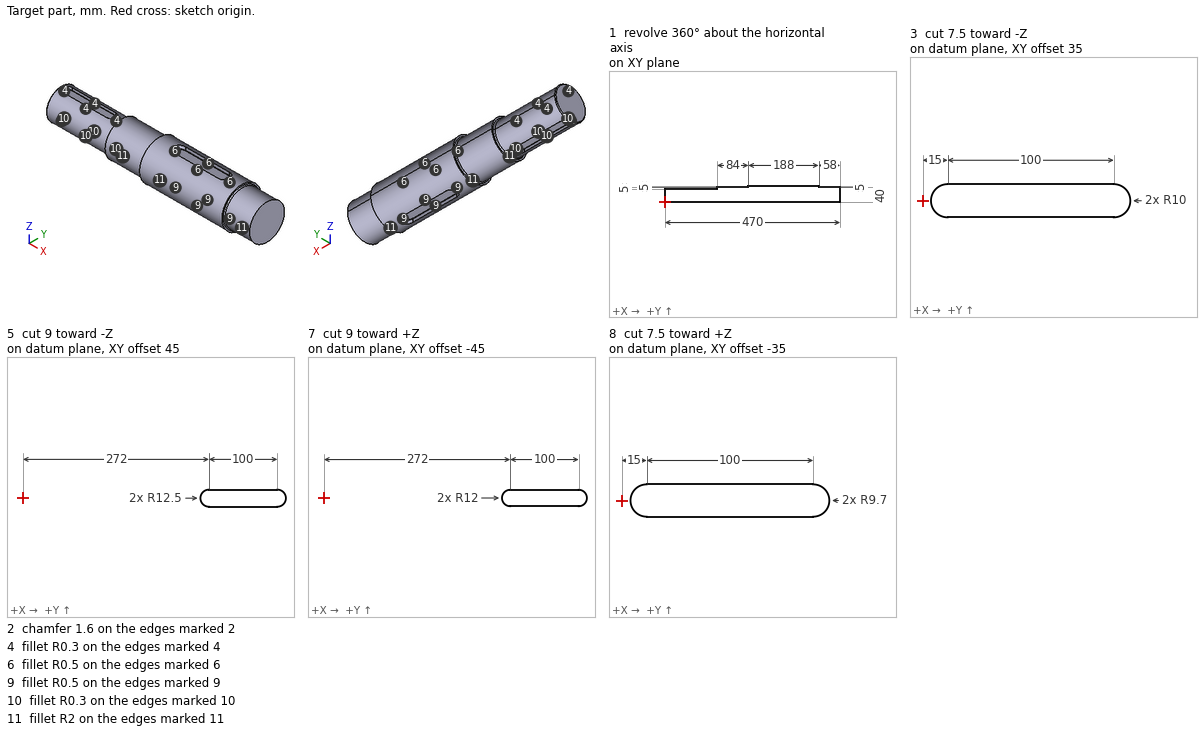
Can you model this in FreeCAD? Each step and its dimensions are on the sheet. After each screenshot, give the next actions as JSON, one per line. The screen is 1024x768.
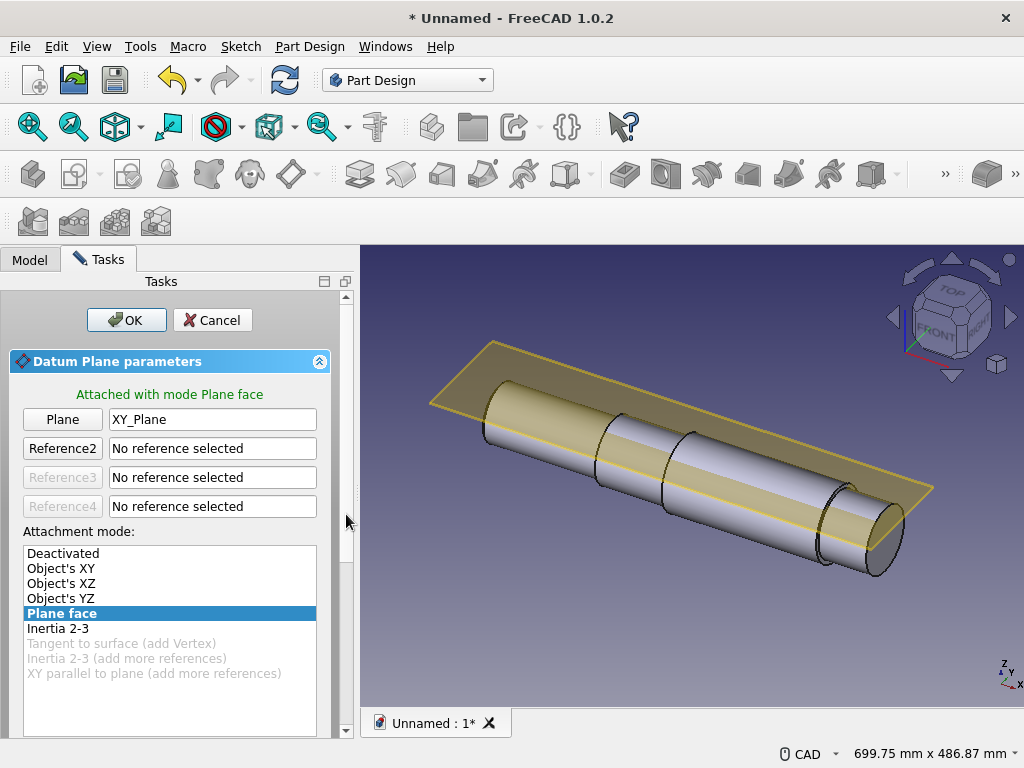
{"action": "left_click", "coordinate": [127, 320]}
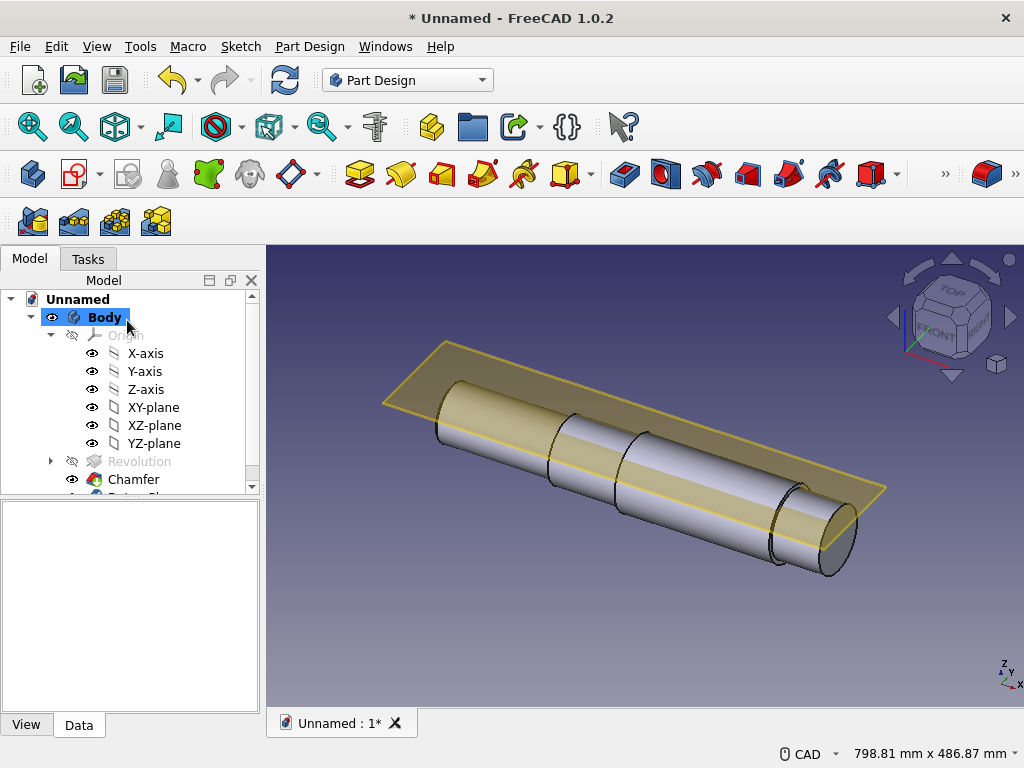
{"action": "scroll", "coordinate": [101, 385], "scroll_direction": "down", "scroll_amount": 3}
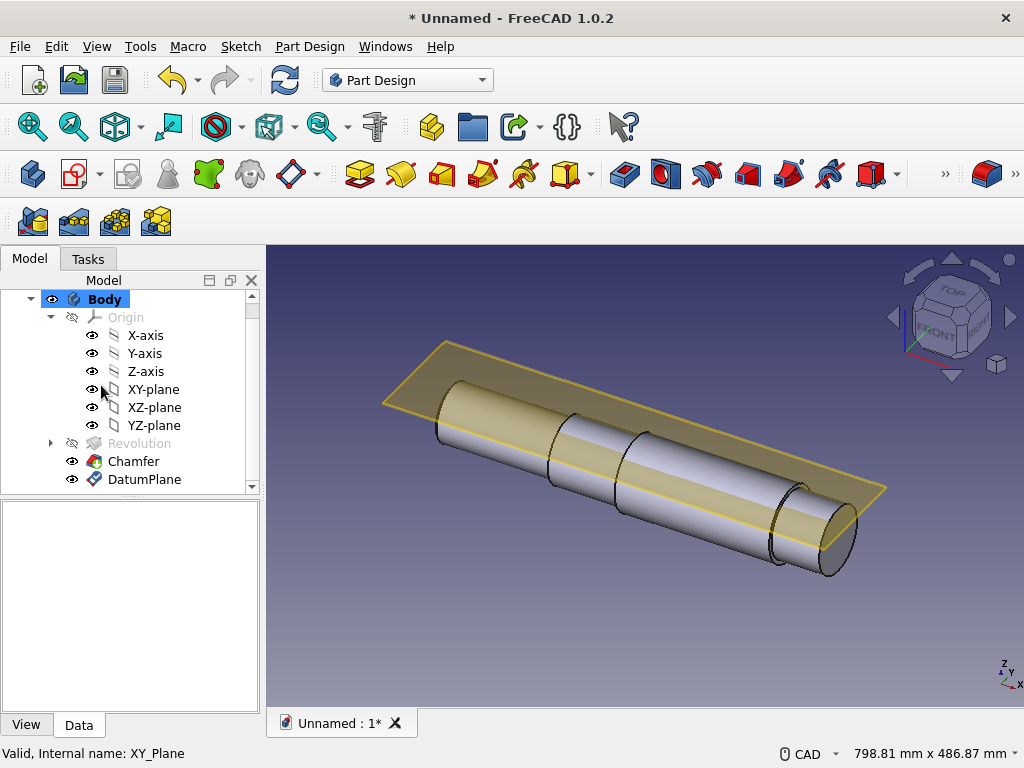
{"action": "left_click", "coordinate": [117, 479]}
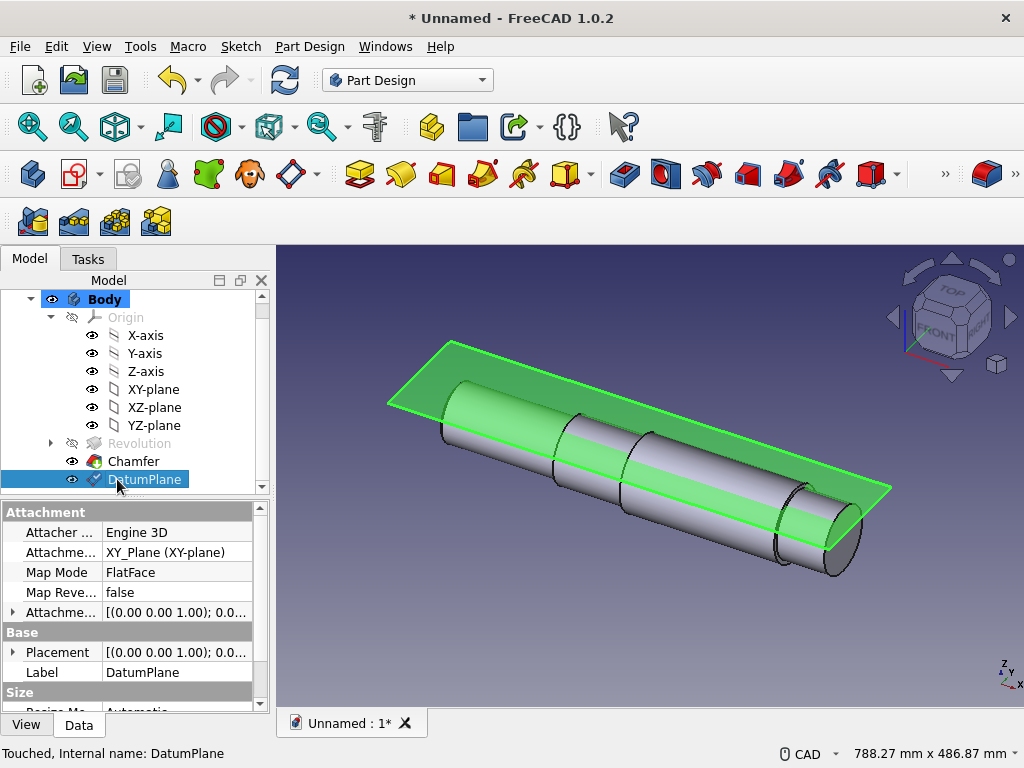
{"action": "left_click", "coordinate": [74, 174]}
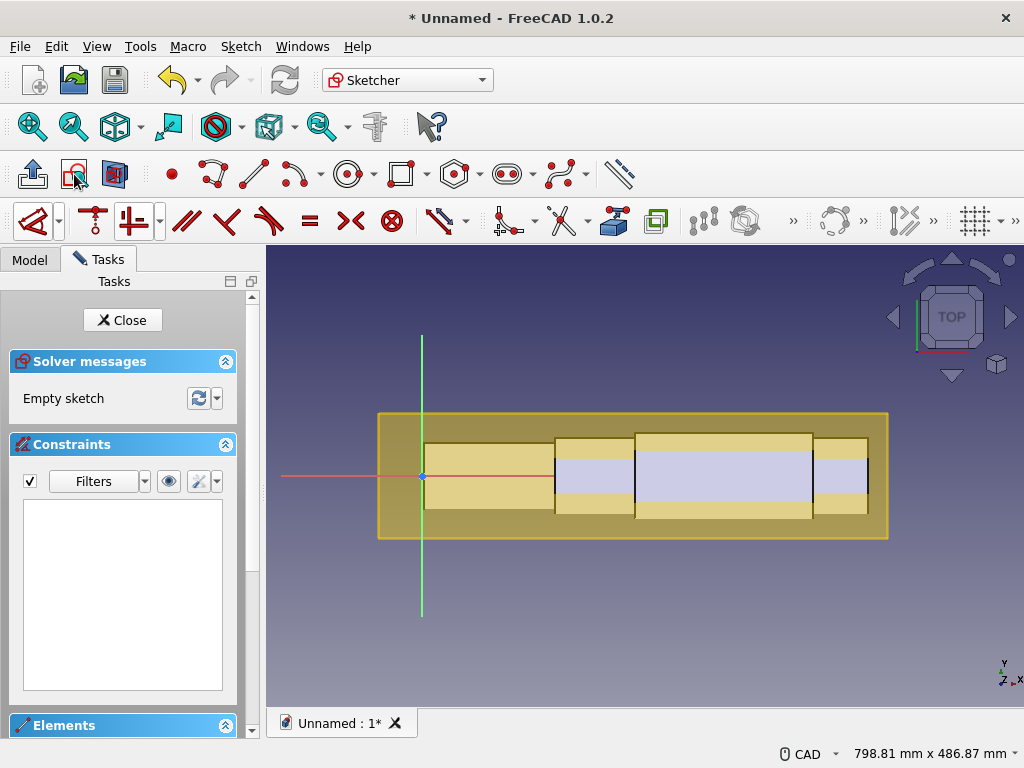
{"action": "left_click", "coordinate": [115, 174]}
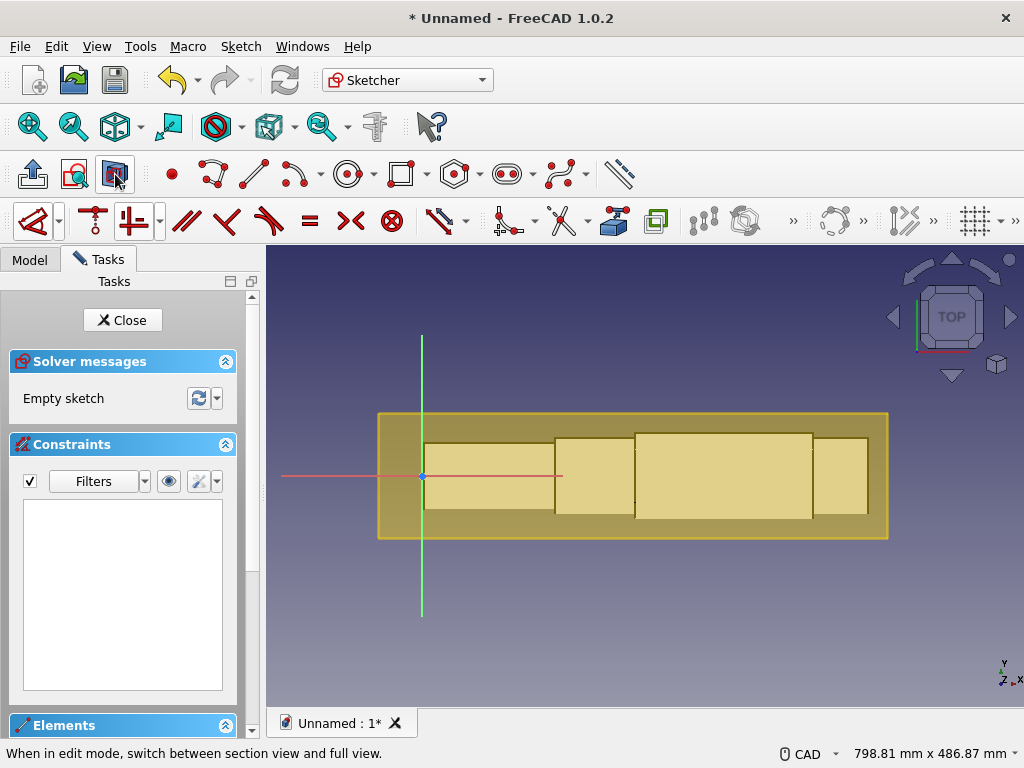
{"action": "scroll", "coordinate": [440, 476], "scroll_direction": "up", "scroll_amount": 6}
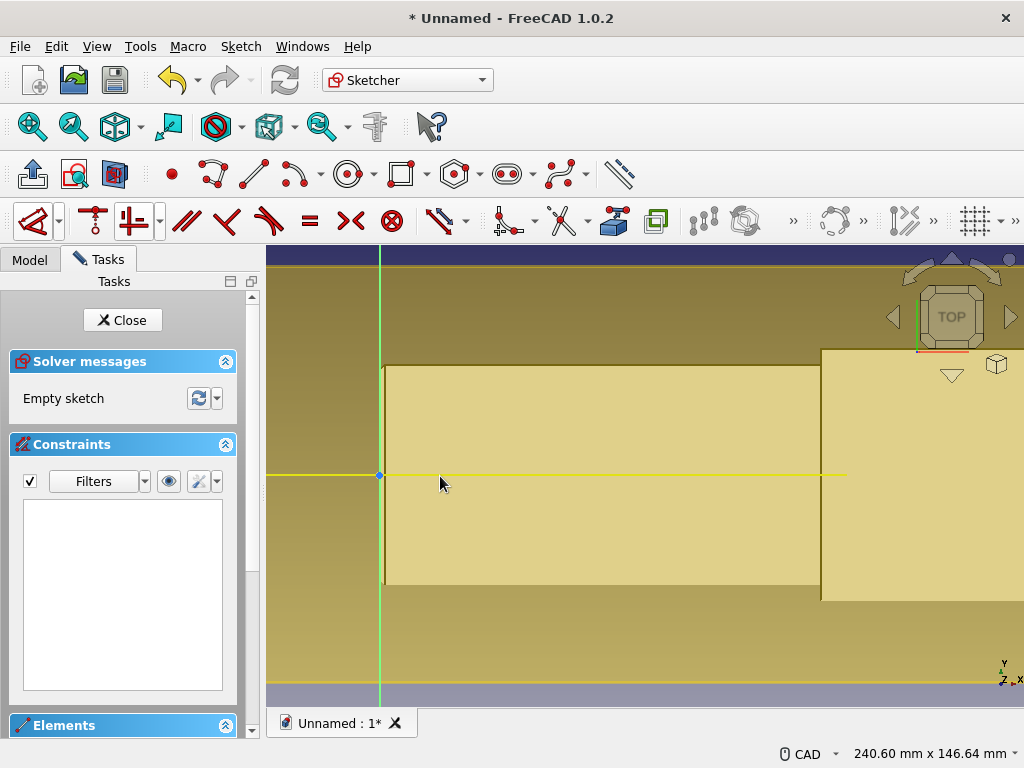
{"action": "left_click", "coordinate": [506, 174]}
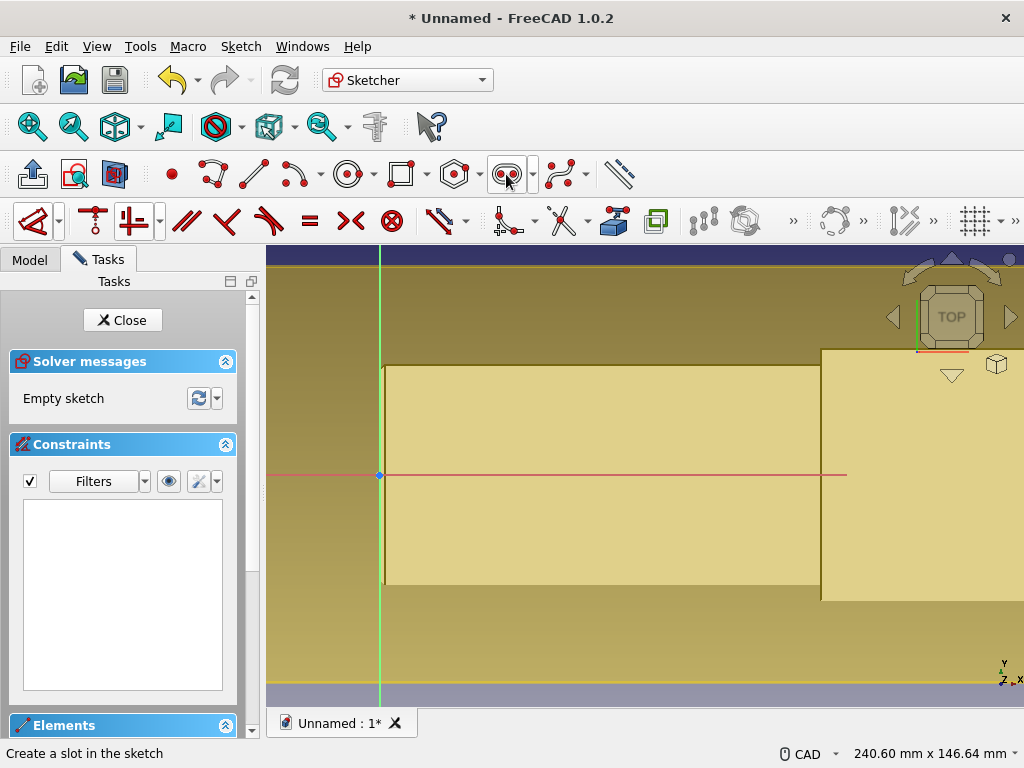
{"action": "left_click", "coordinate": [427, 475]}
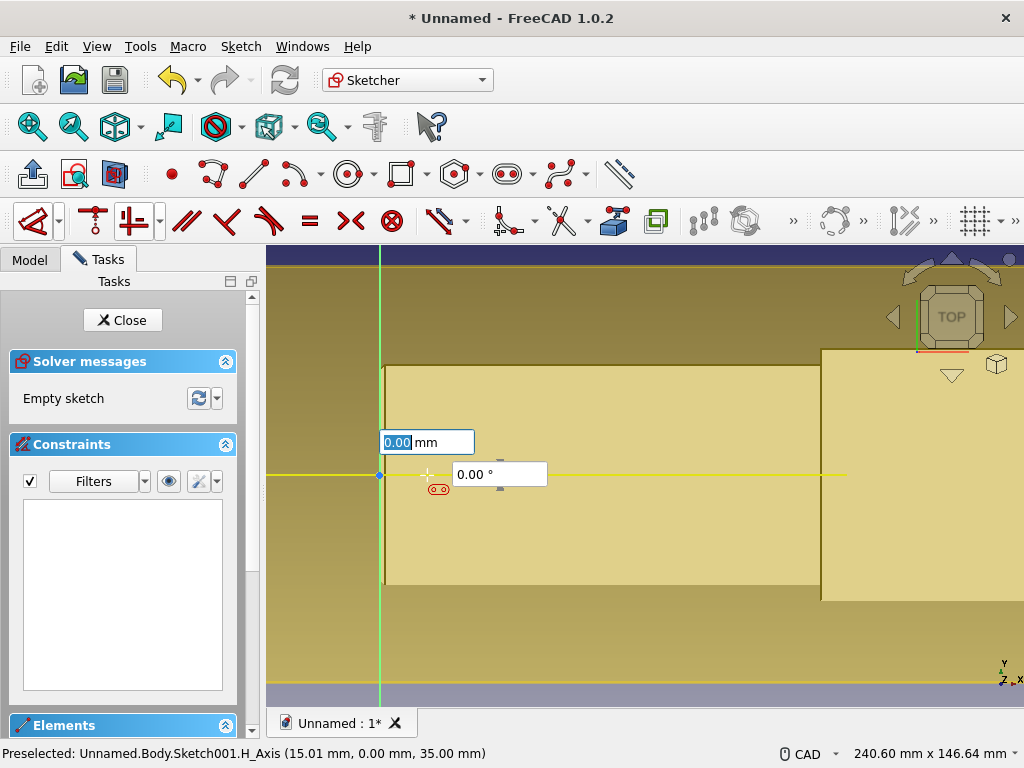
{"action": "left_click", "coordinate": [742, 466]}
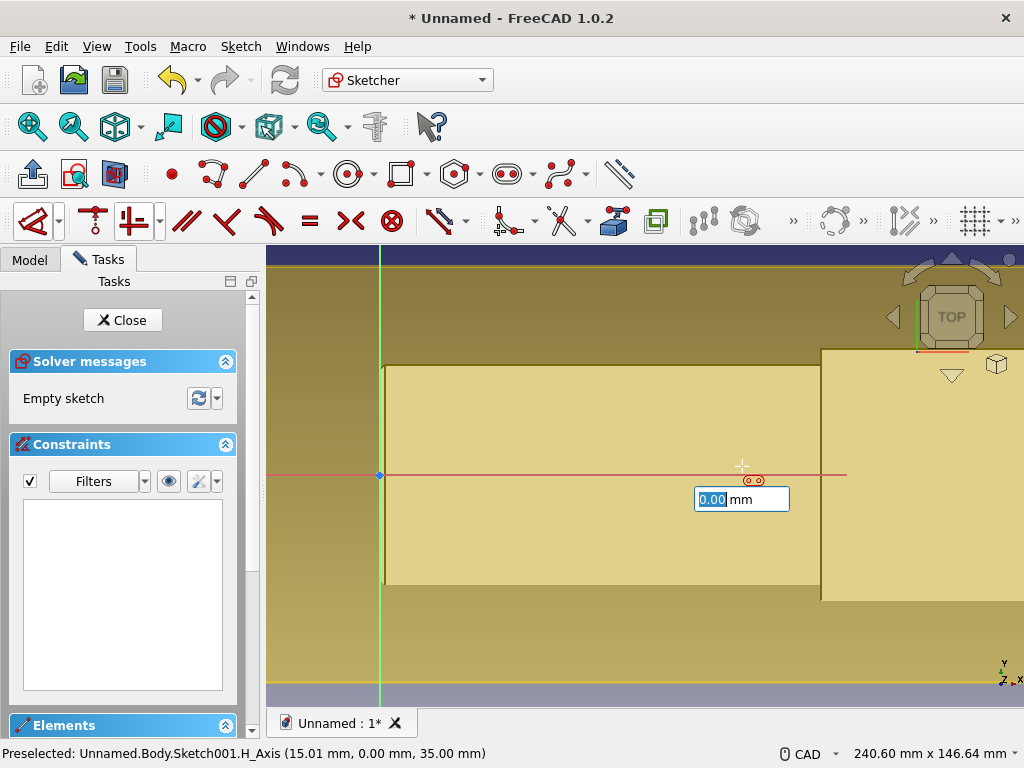
{"action": "left_click", "coordinate": [585, 444]}
{"action": "key", "text": "Escape"}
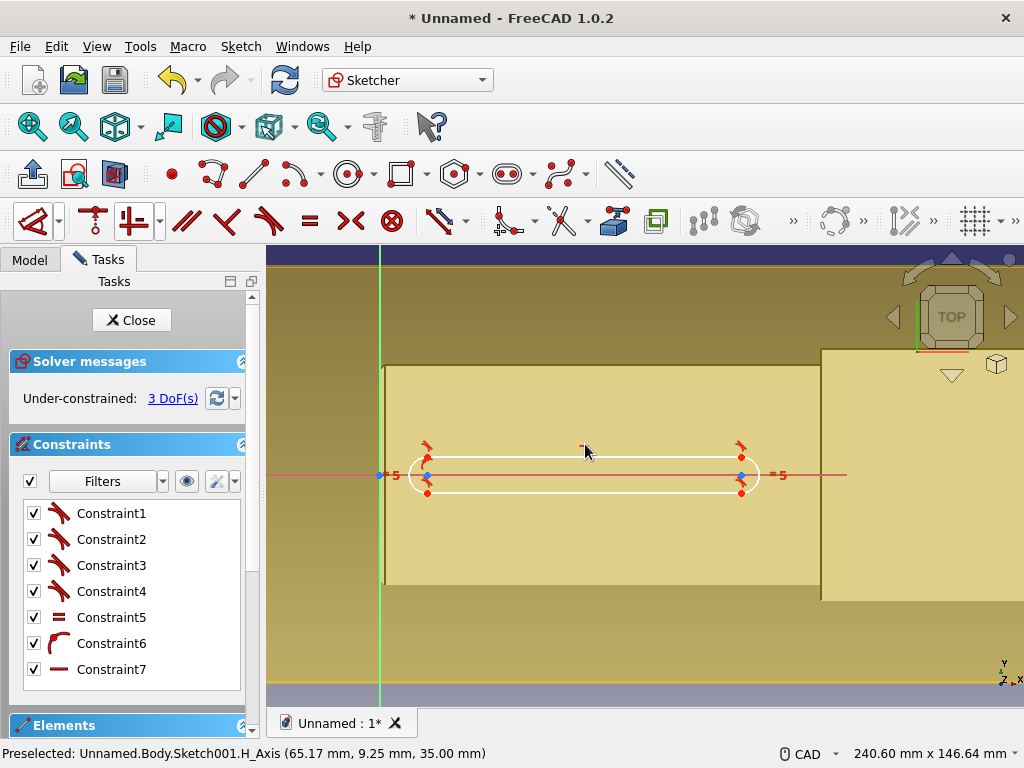
{"action": "scroll", "coordinate": [413, 465], "scroll_direction": "up", "scroll_amount": 2}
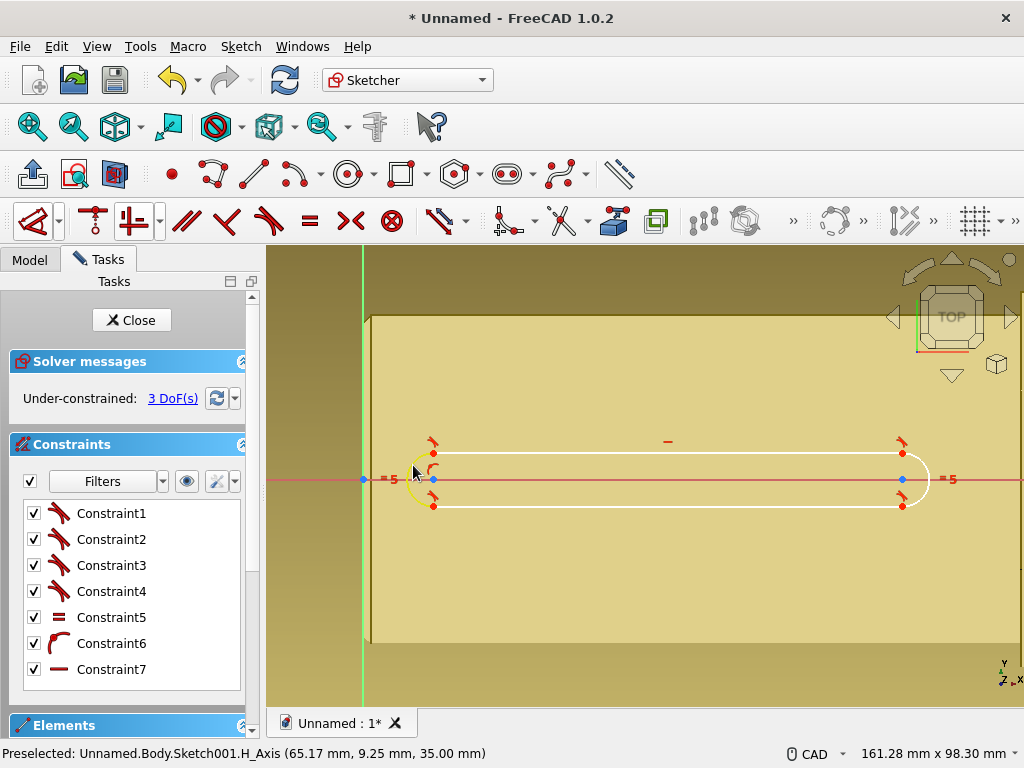
{"action": "left_click", "coordinate": [412, 464]}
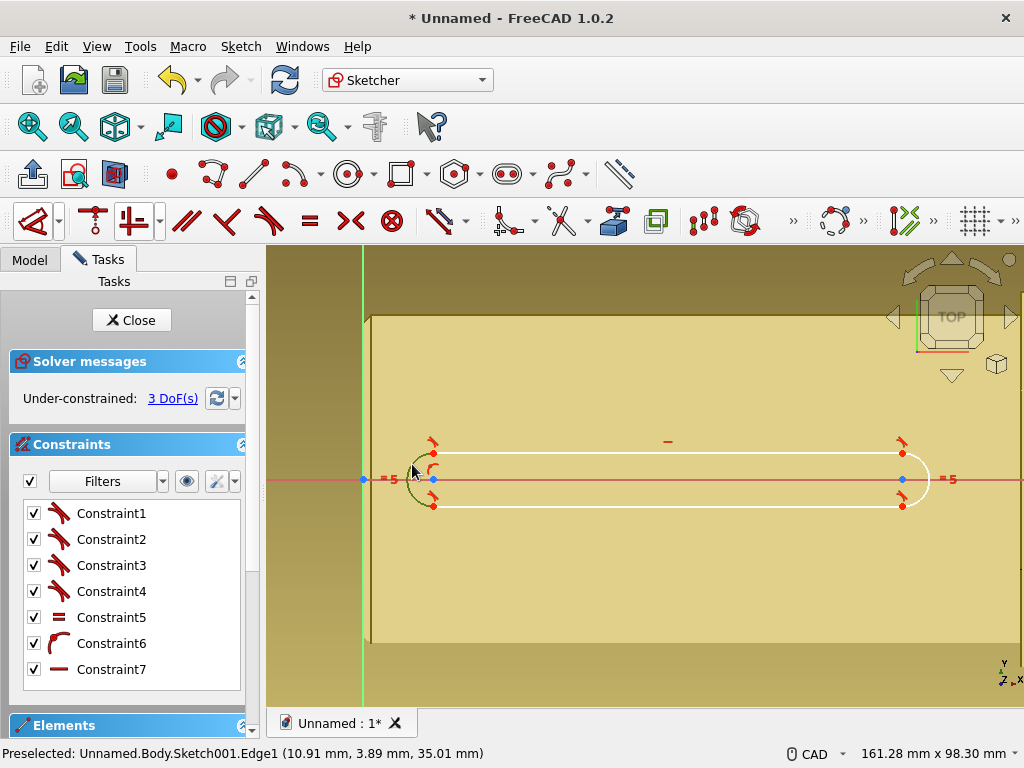
{"action": "left_click", "coordinate": [58, 222]}